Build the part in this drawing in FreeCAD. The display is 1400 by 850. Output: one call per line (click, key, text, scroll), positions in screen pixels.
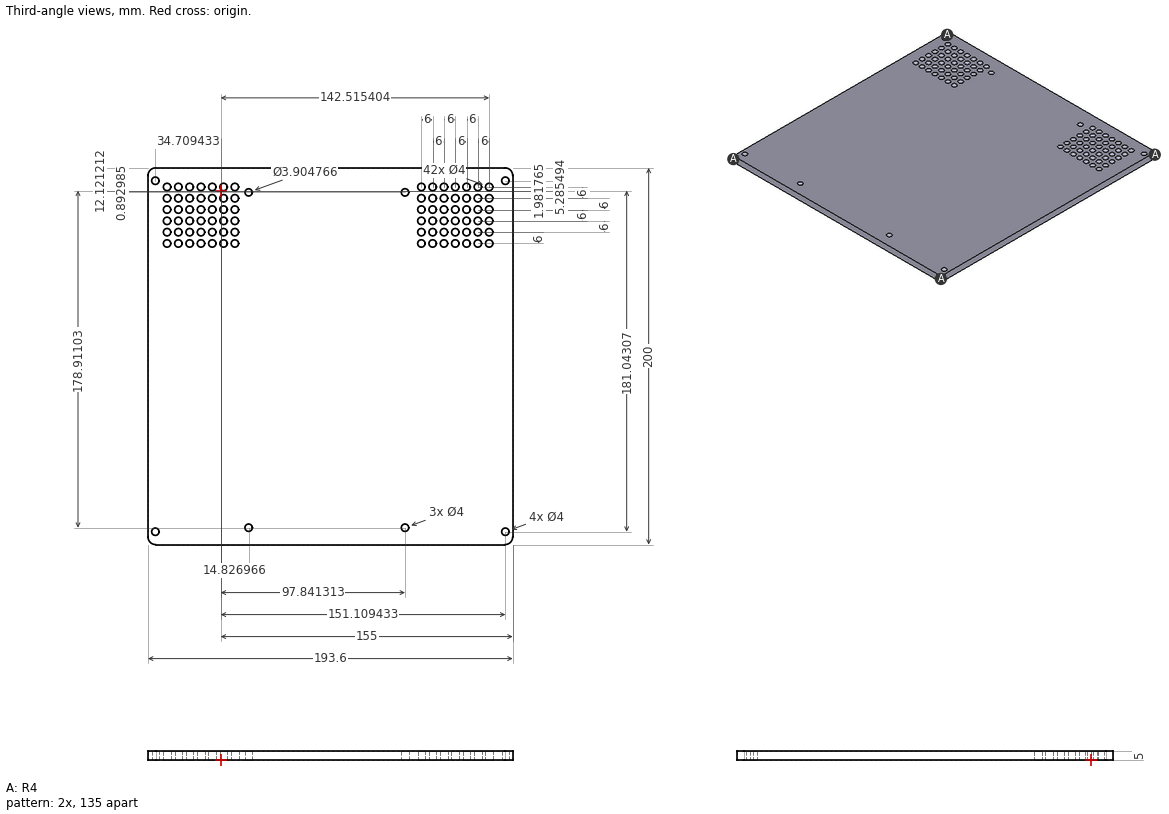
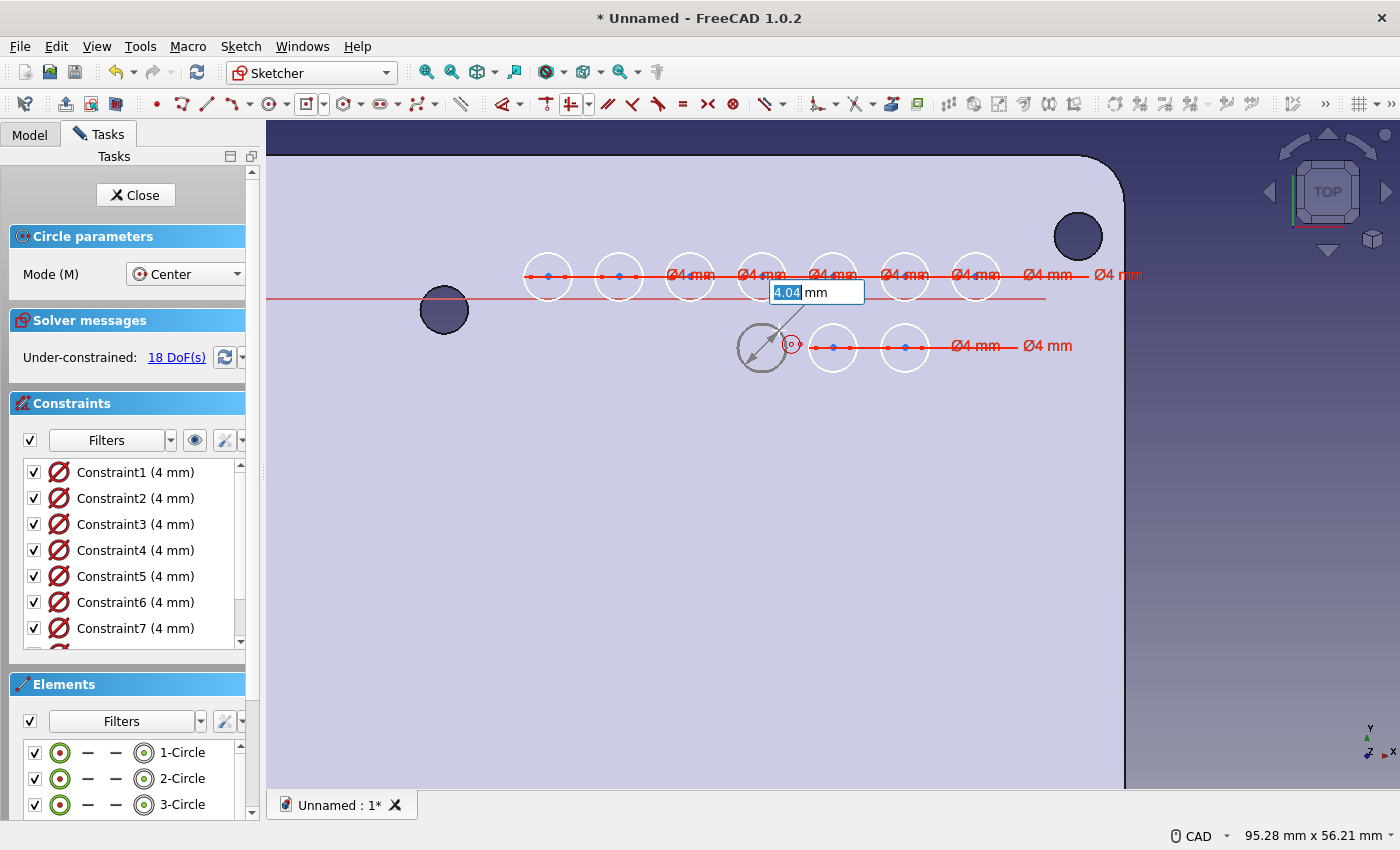
text(4)
key(Return)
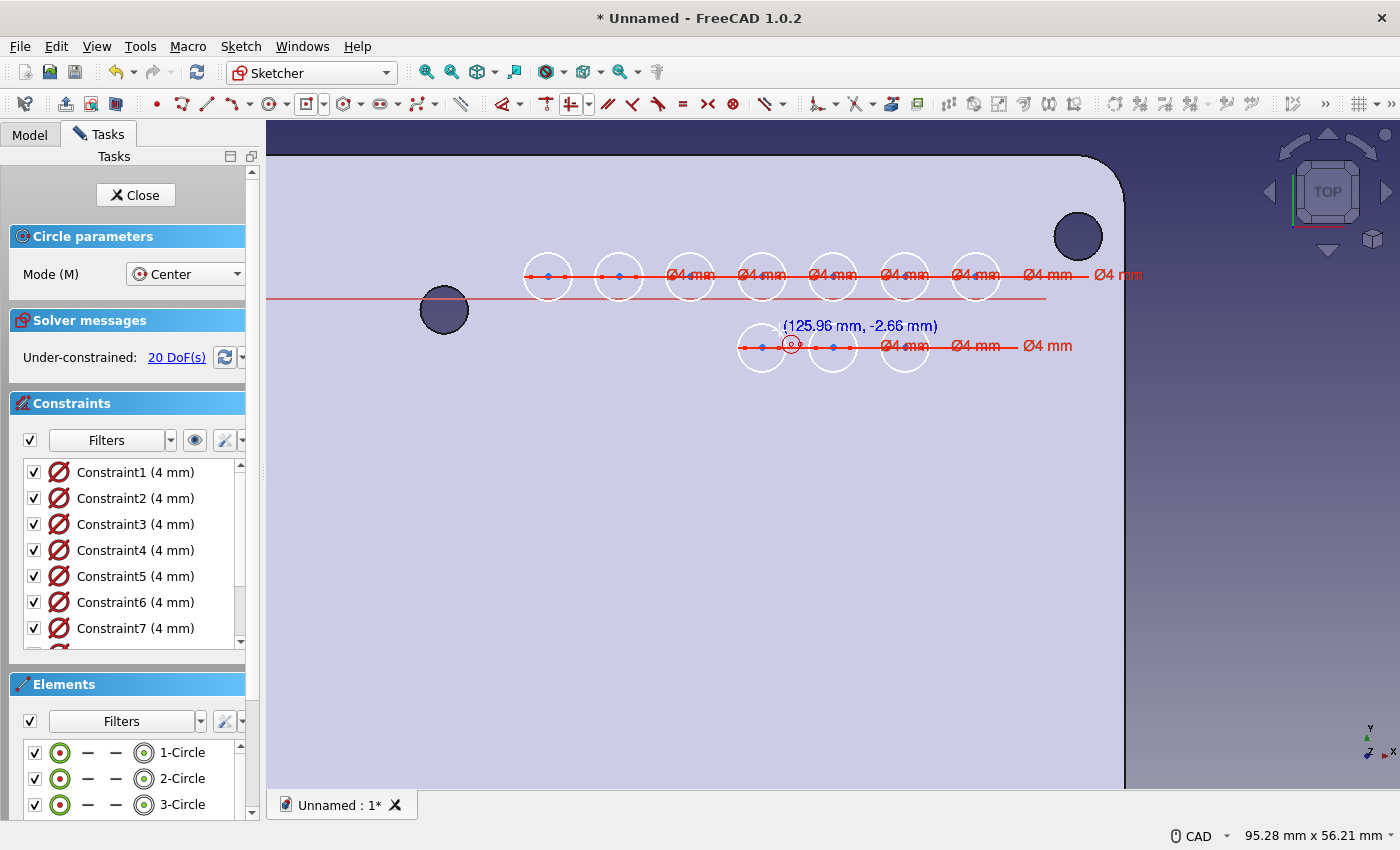
click(690, 347)
move(707, 330)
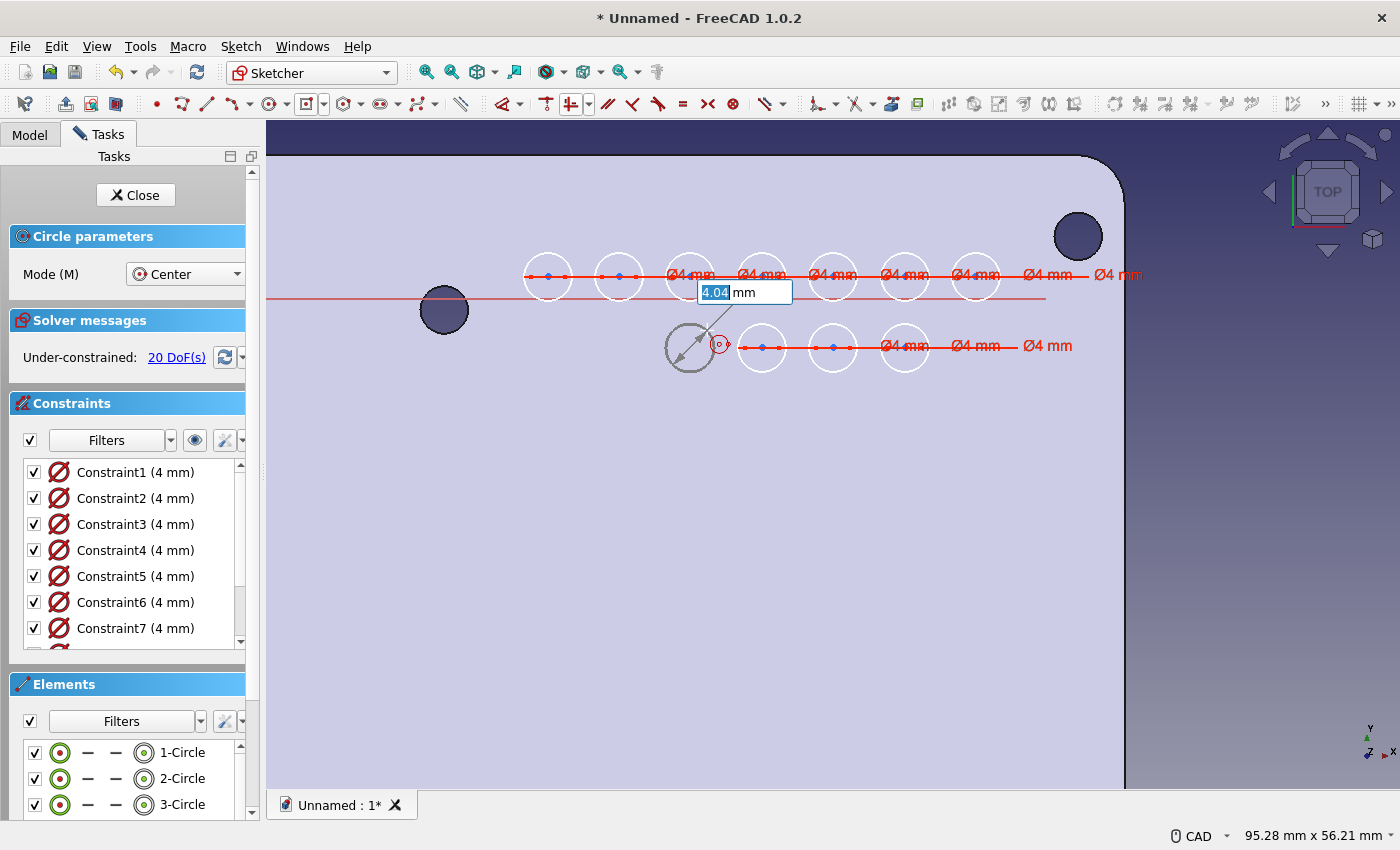
text(4)
key(Return)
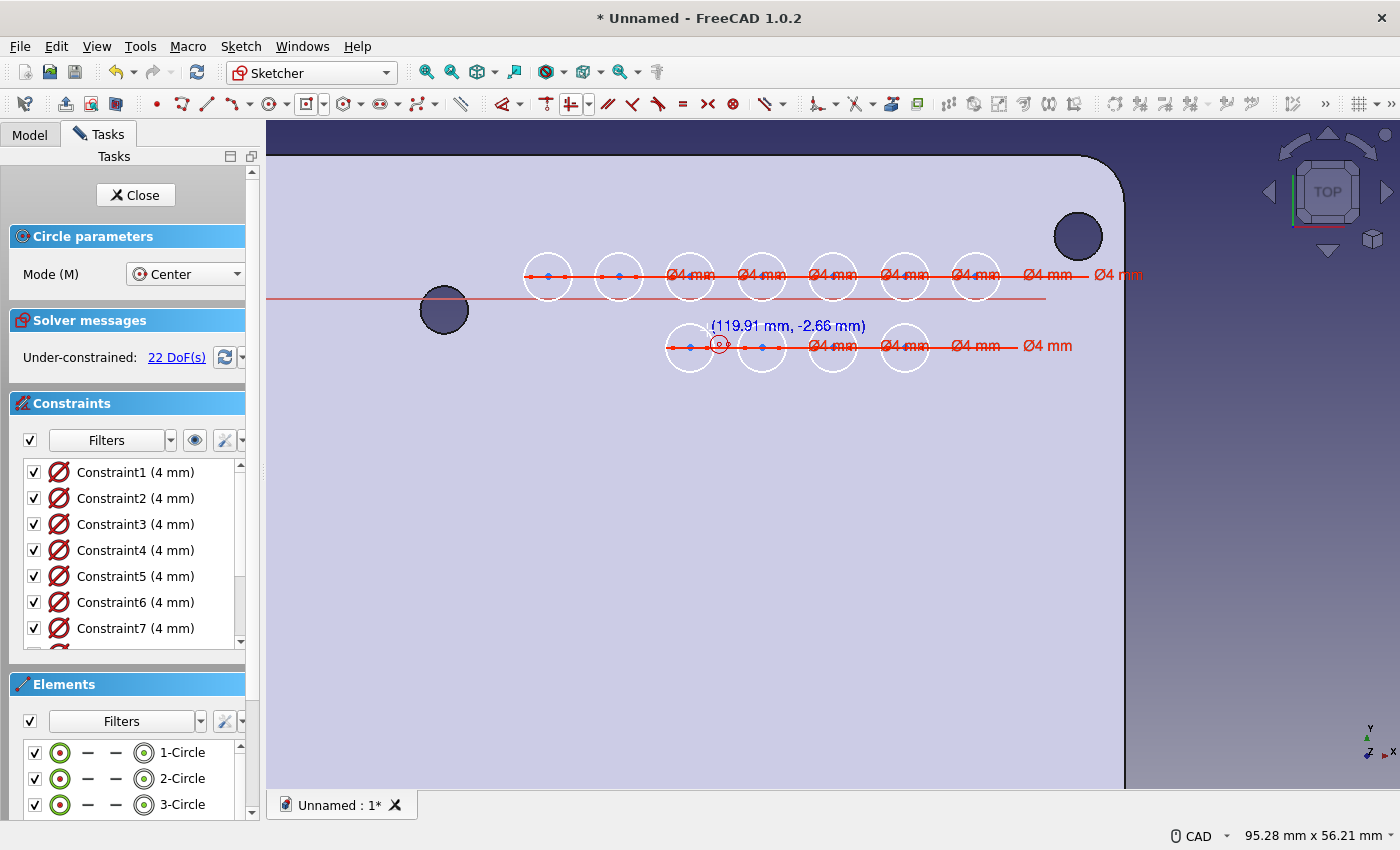
click(619, 347)
move(636, 330)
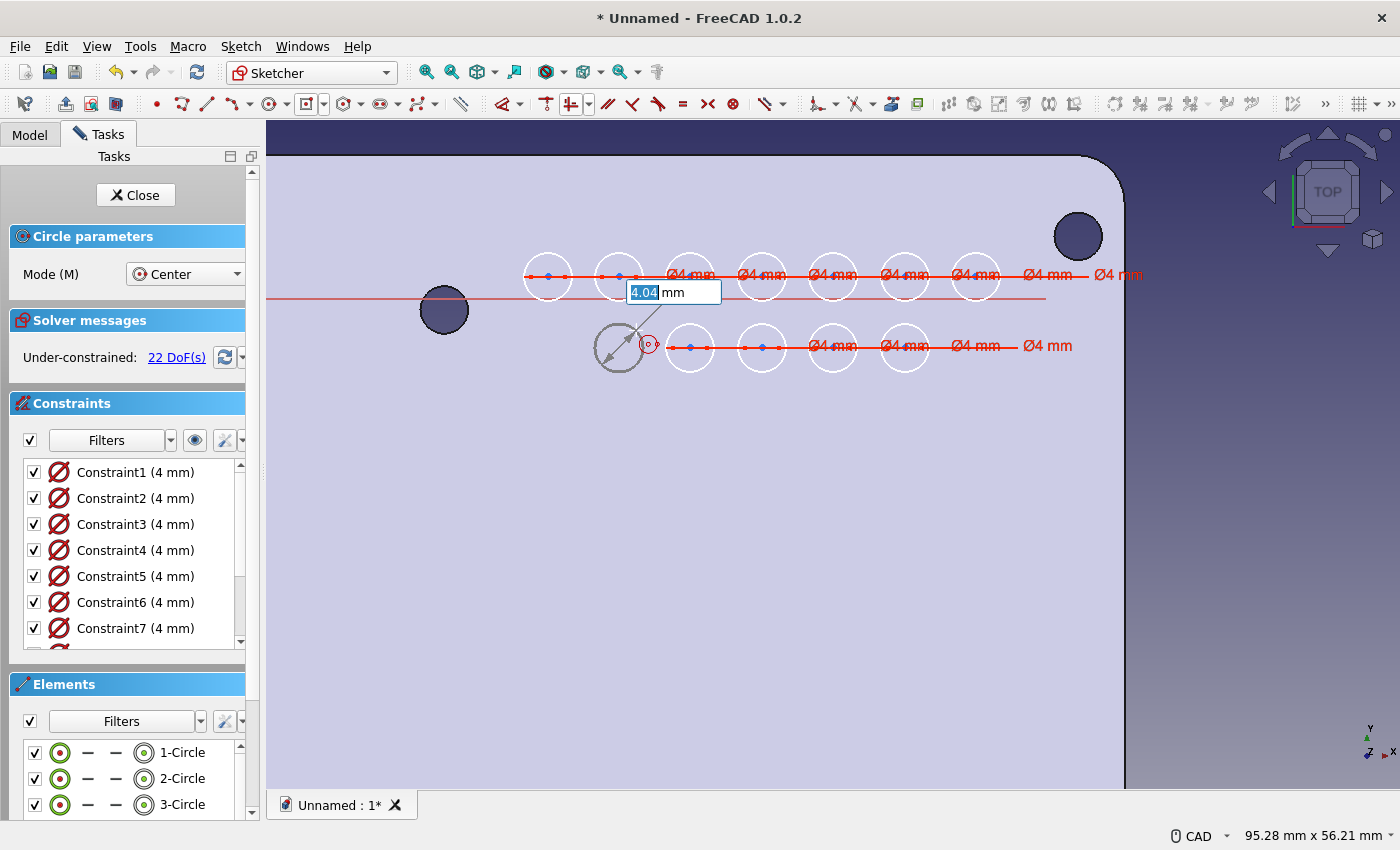
text(4)
key(Return)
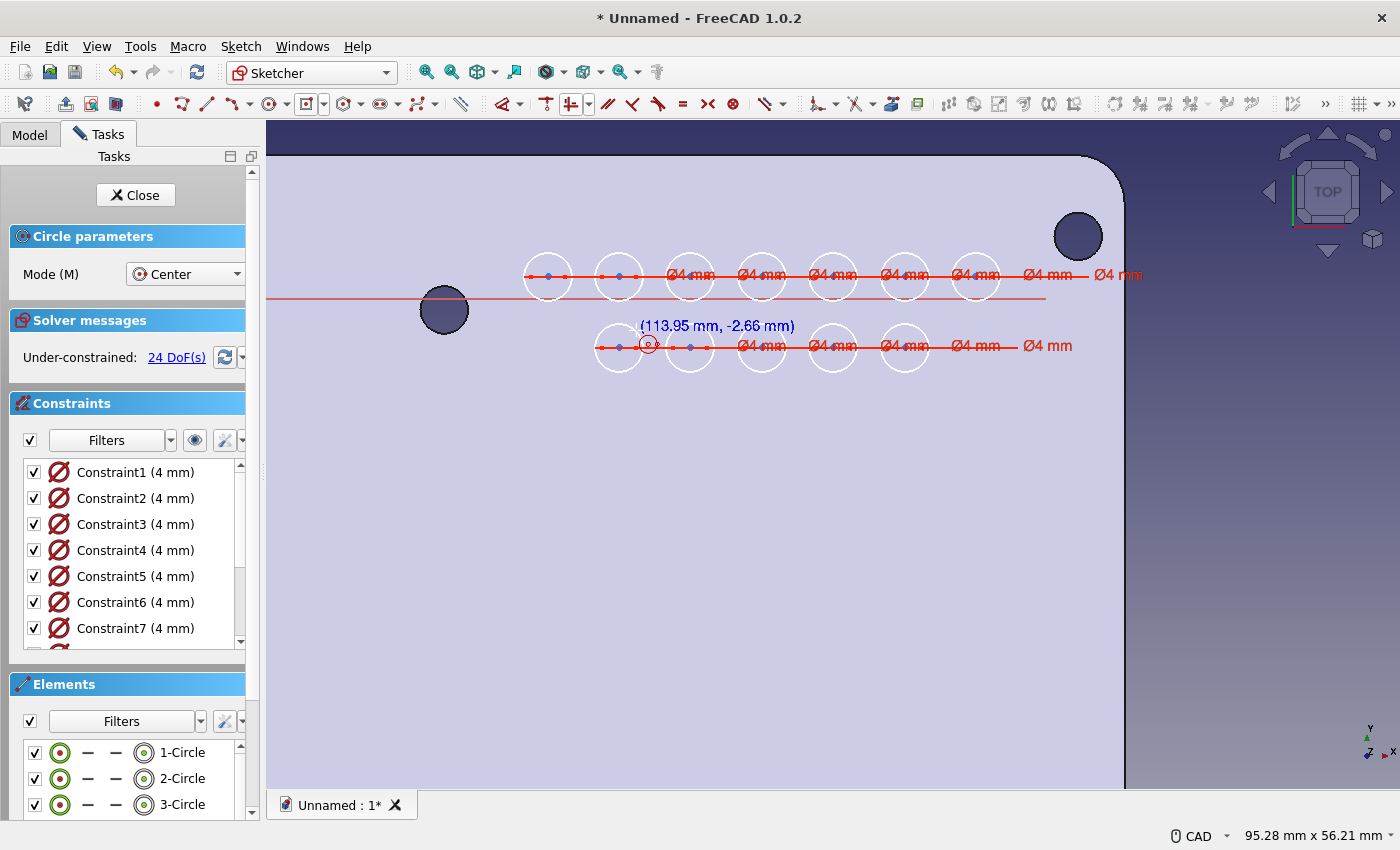
click(548, 347)
move(564, 330)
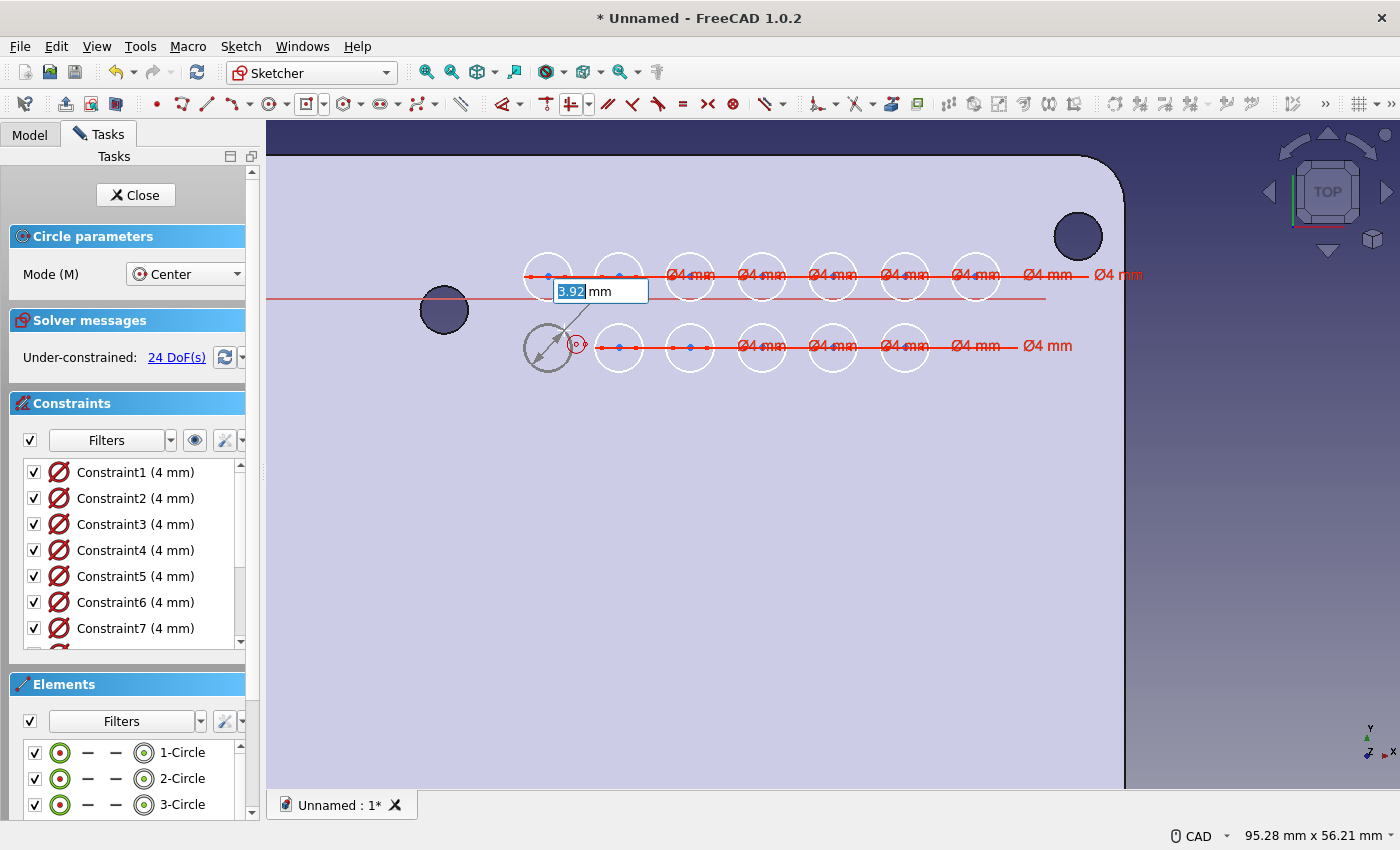
text(4)
key(Return)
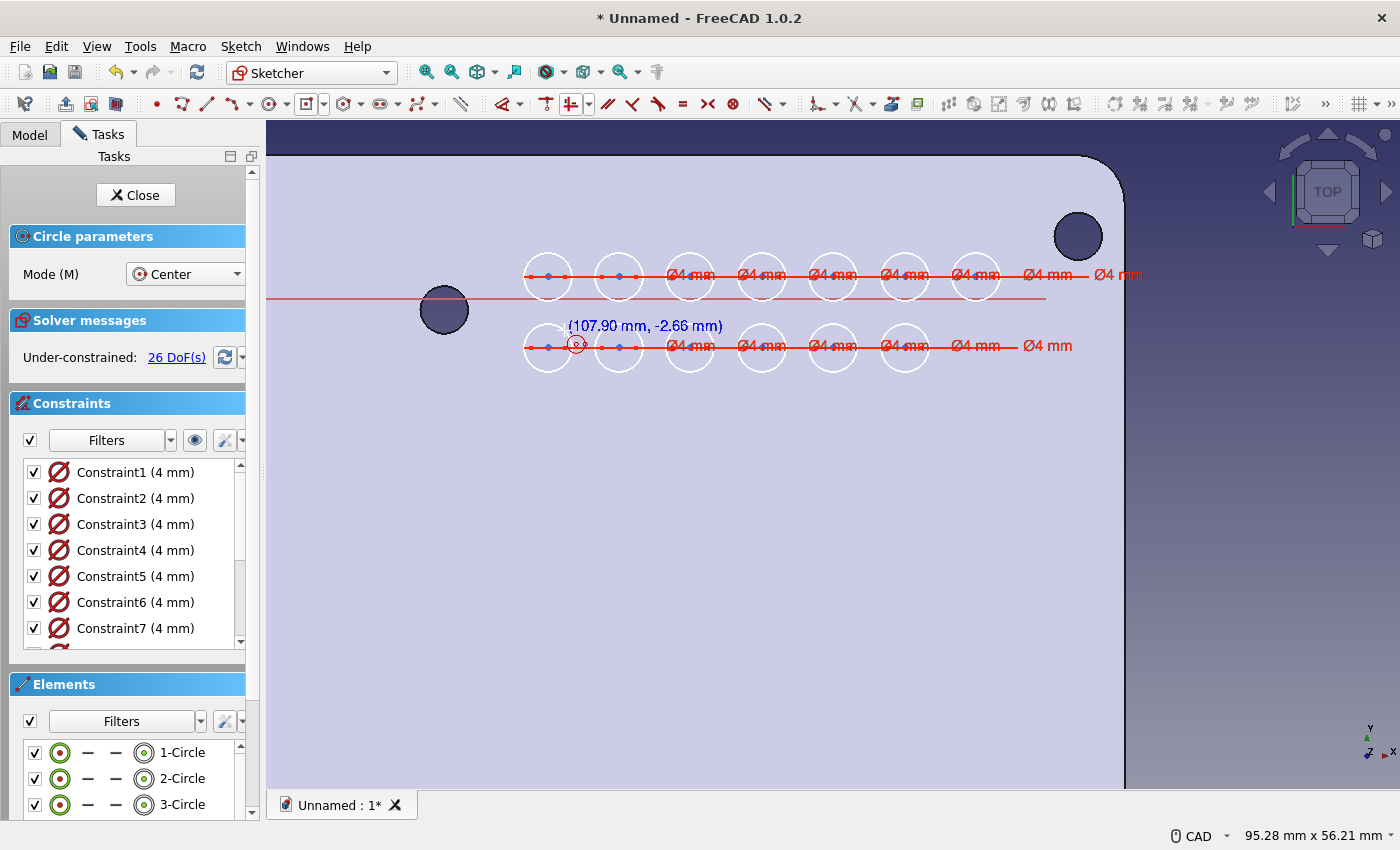
click(905, 419)
move(921, 402)